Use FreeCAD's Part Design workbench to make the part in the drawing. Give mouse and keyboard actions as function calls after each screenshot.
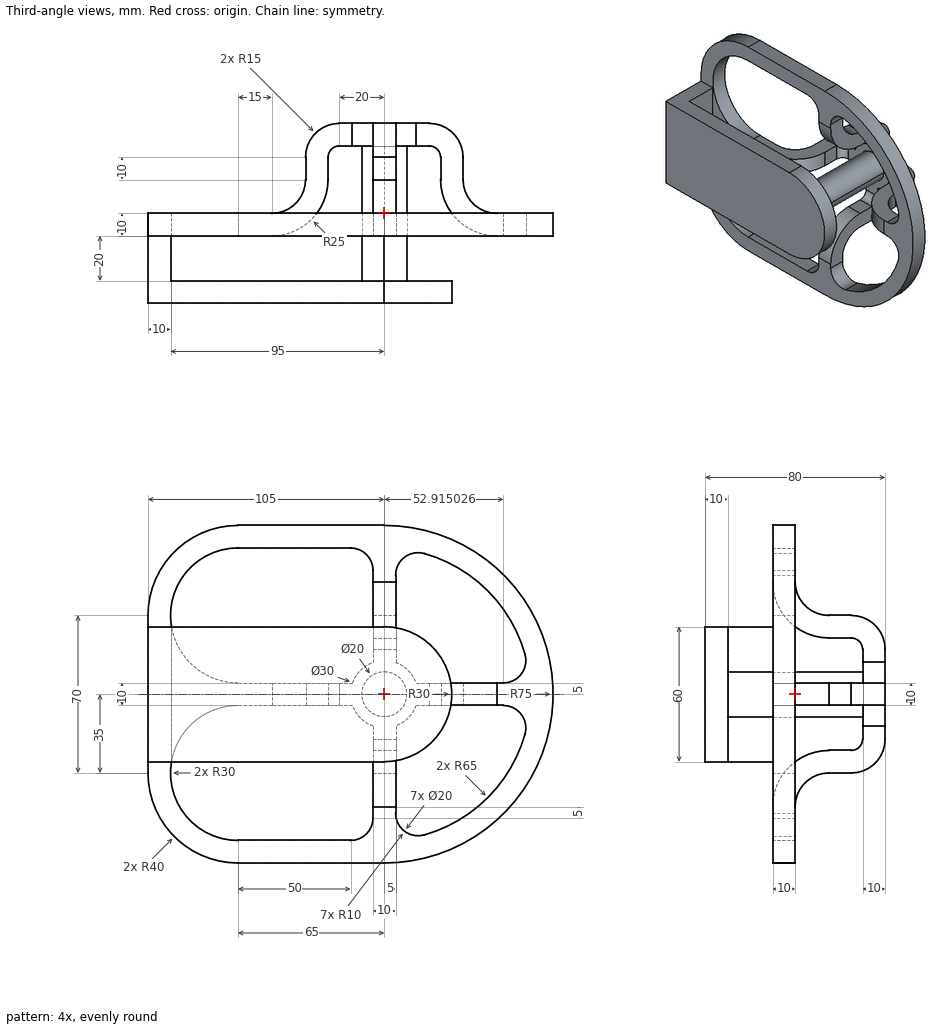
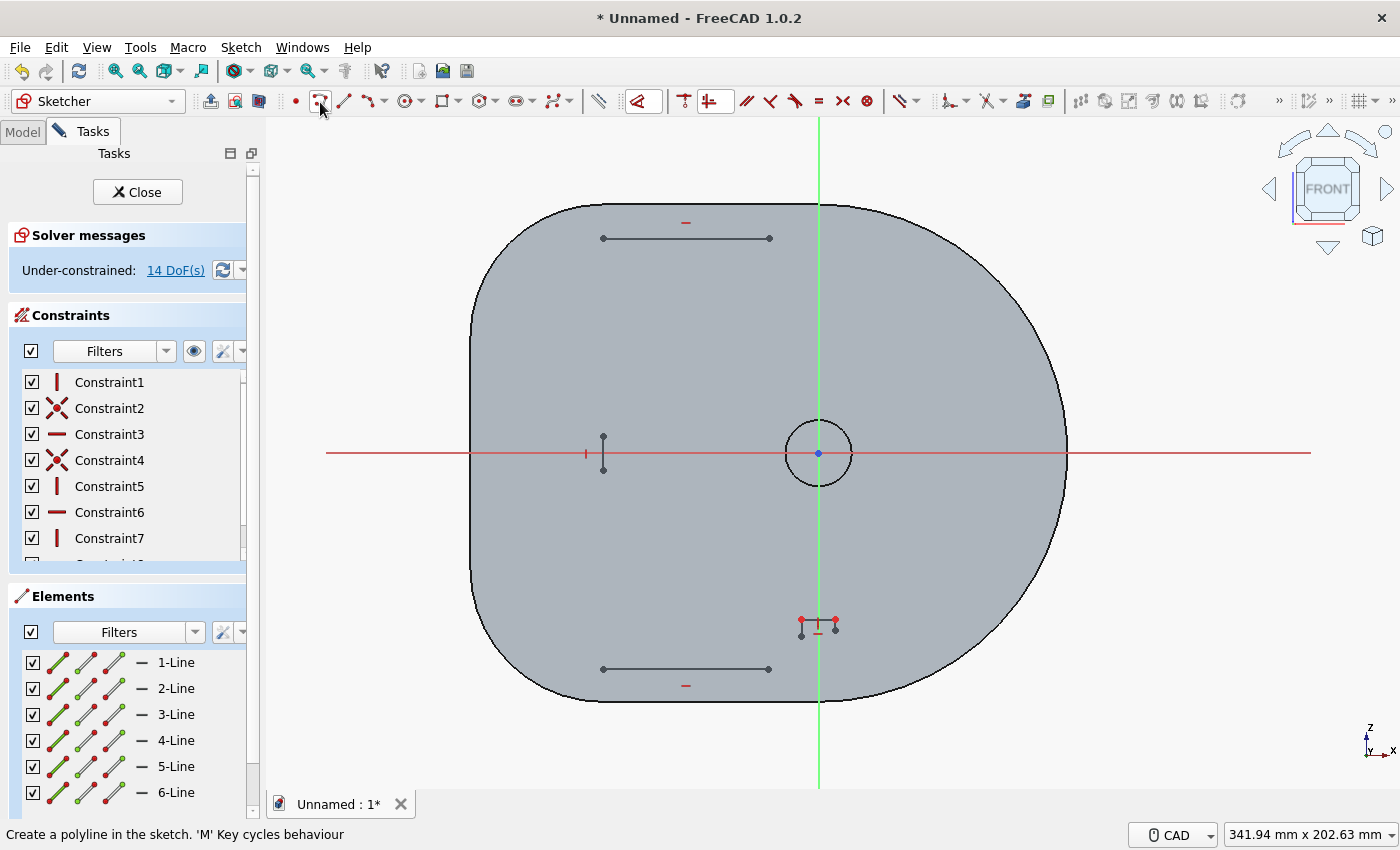
click(802, 271)
click(802, 287)
click(835, 287)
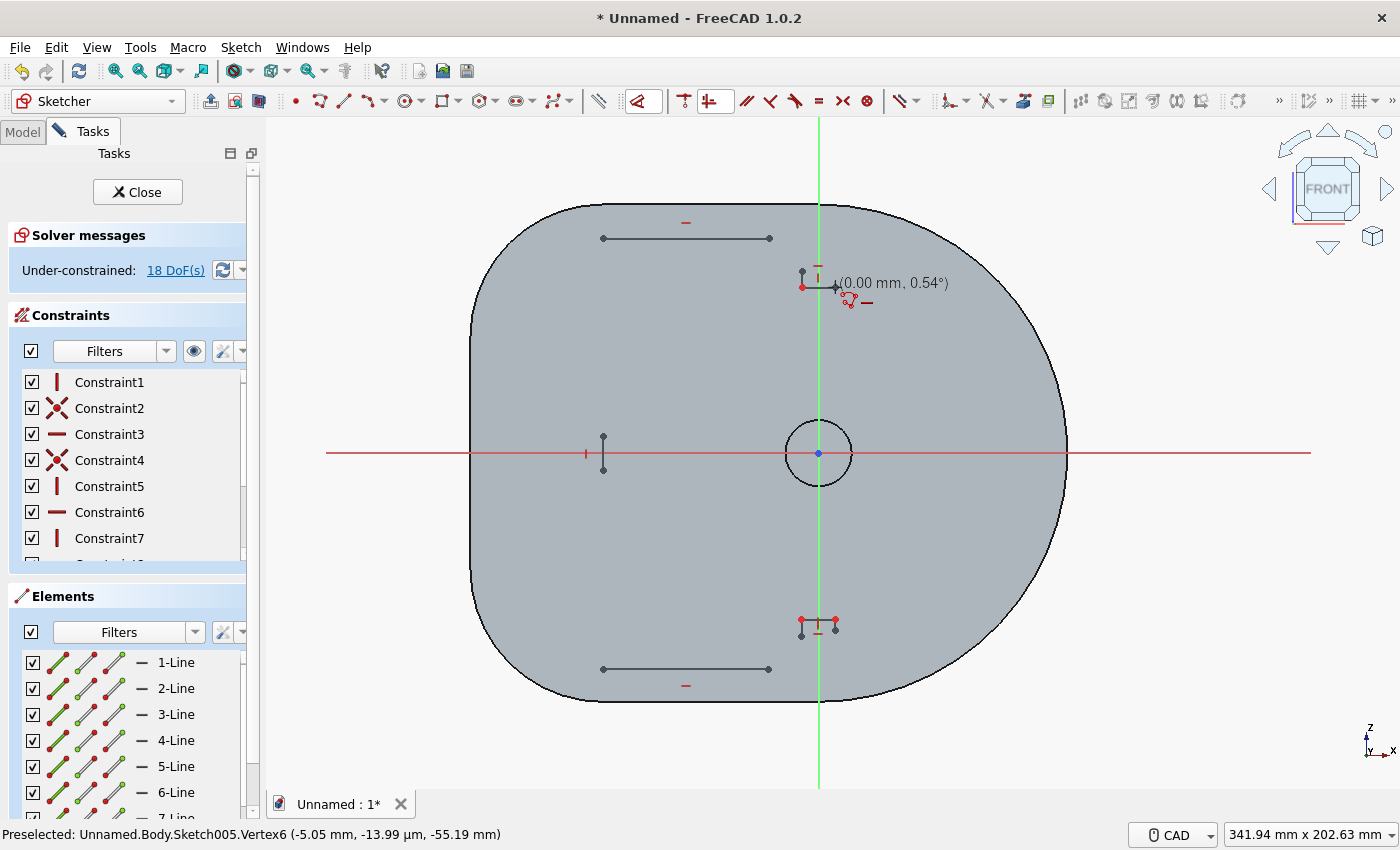
scroll(835, 278, up, 3)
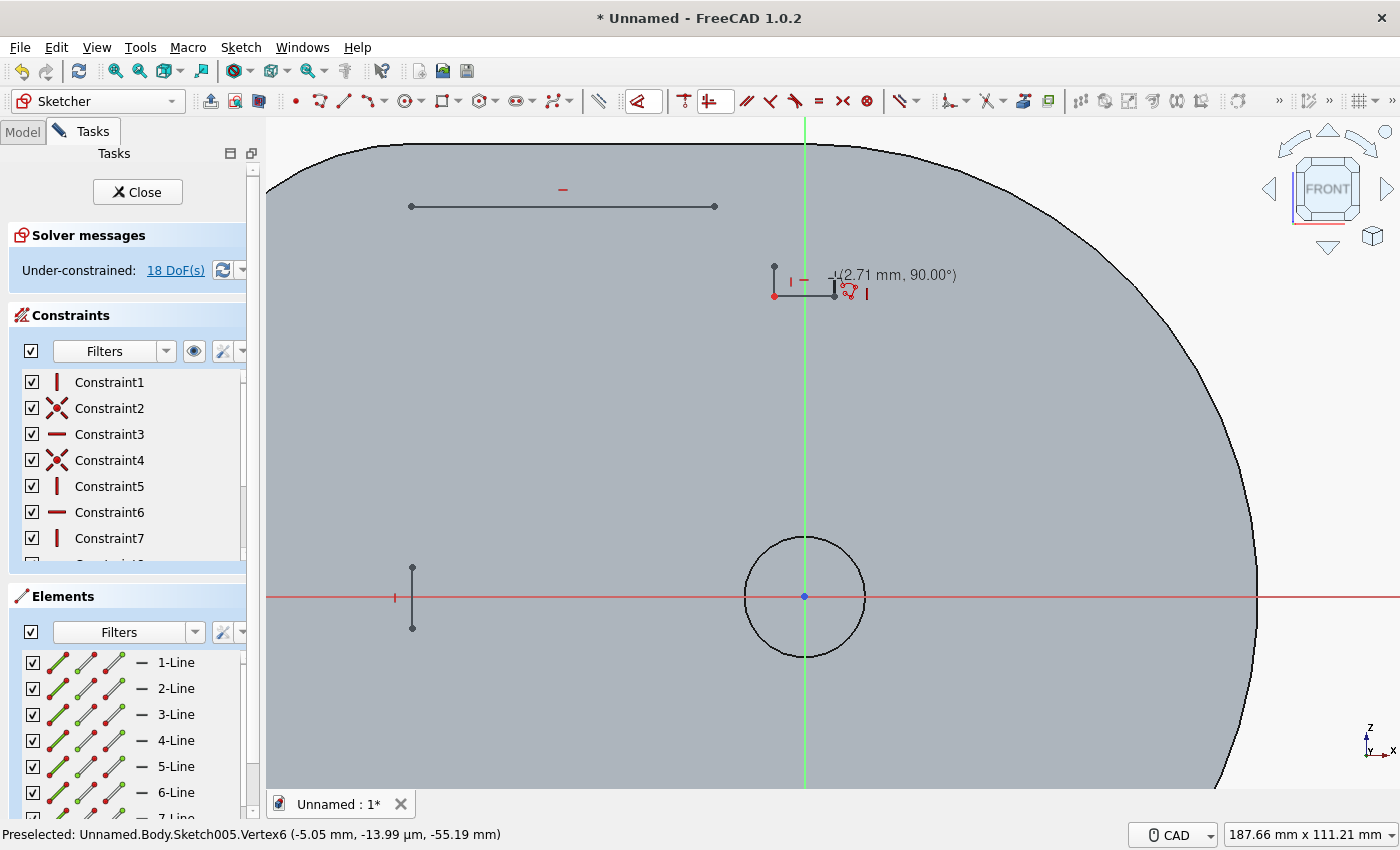
click(835, 277)
right_click(835, 277)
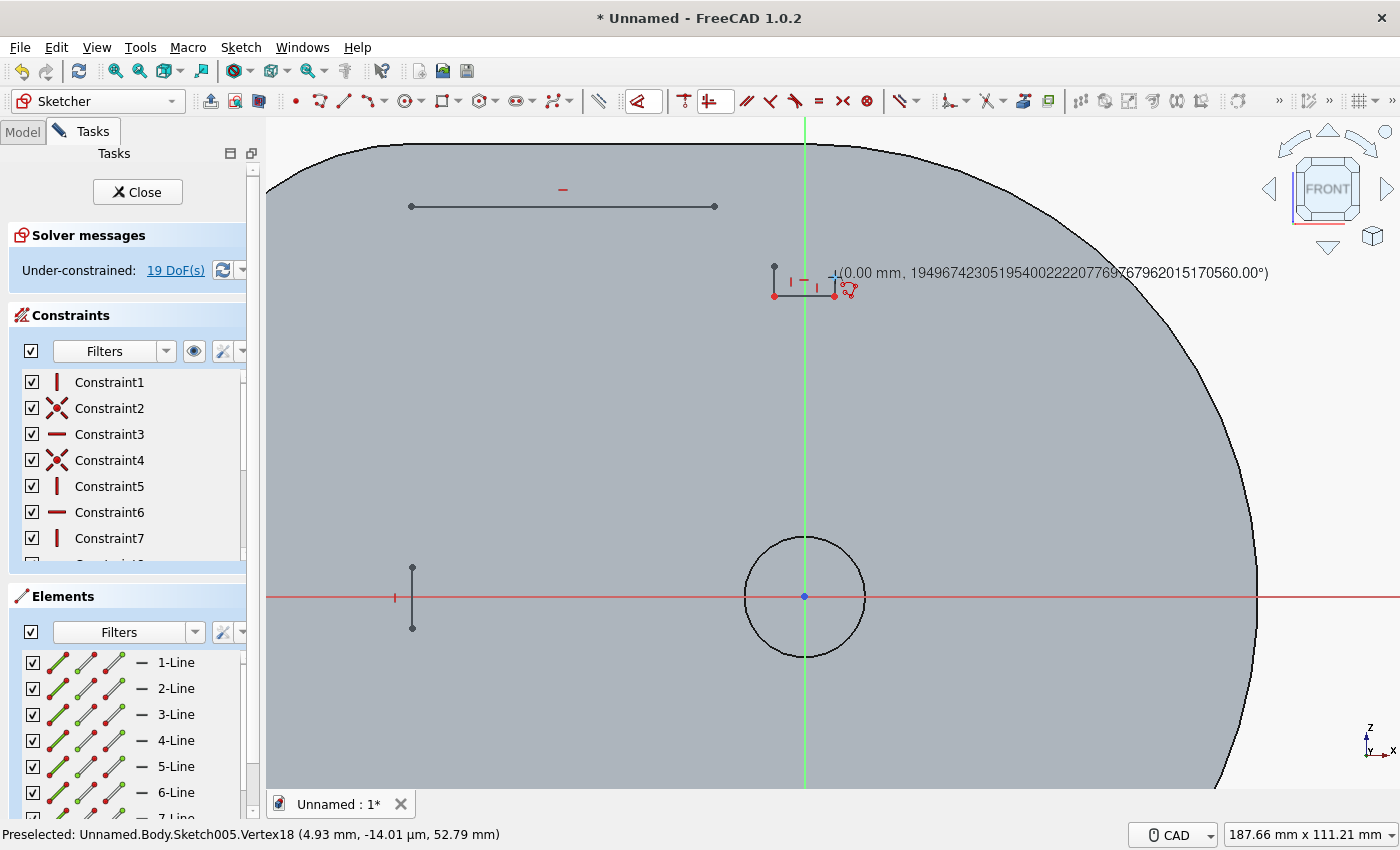
click(344, 102)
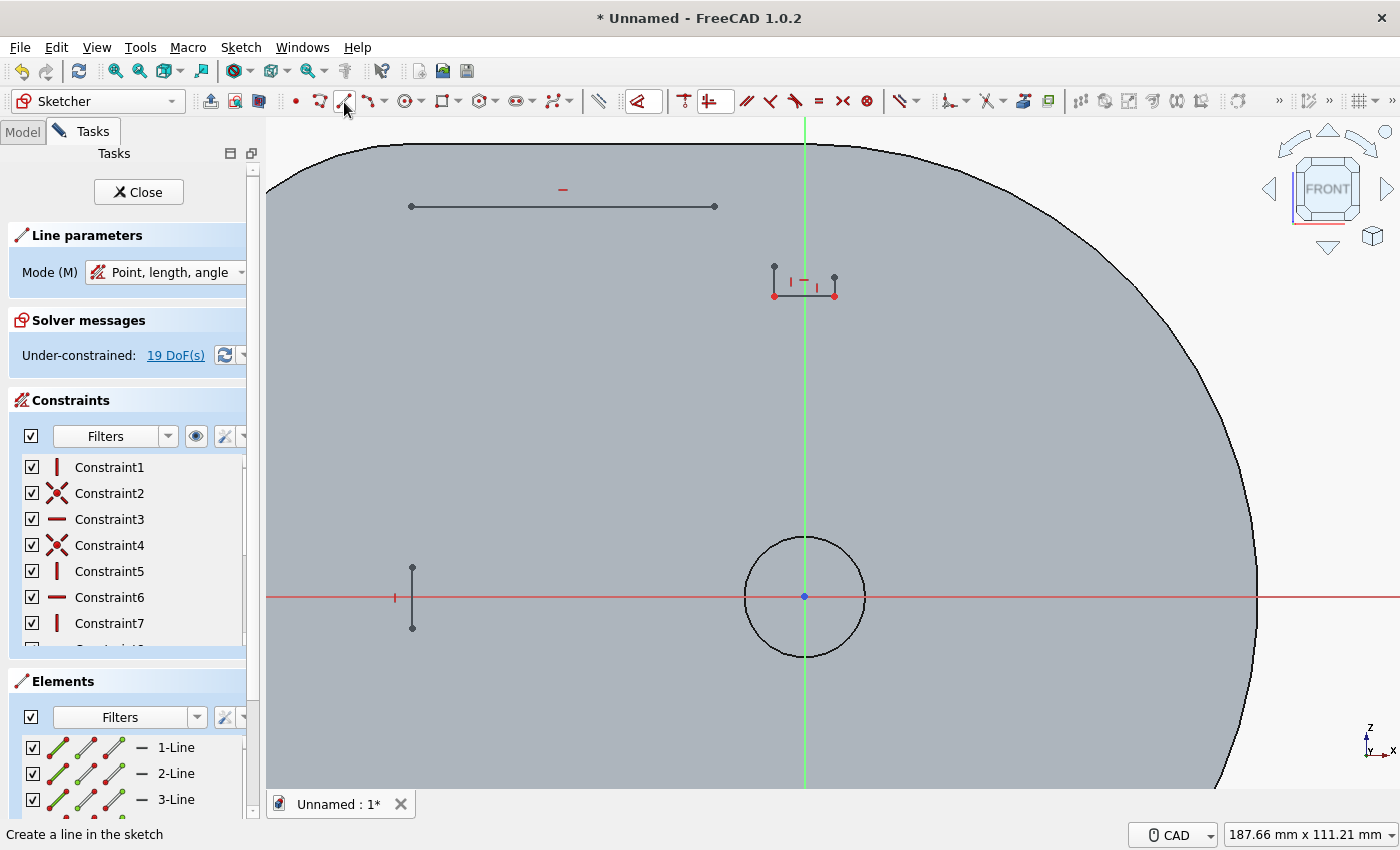
click(1125, 567)
click(1125, 627)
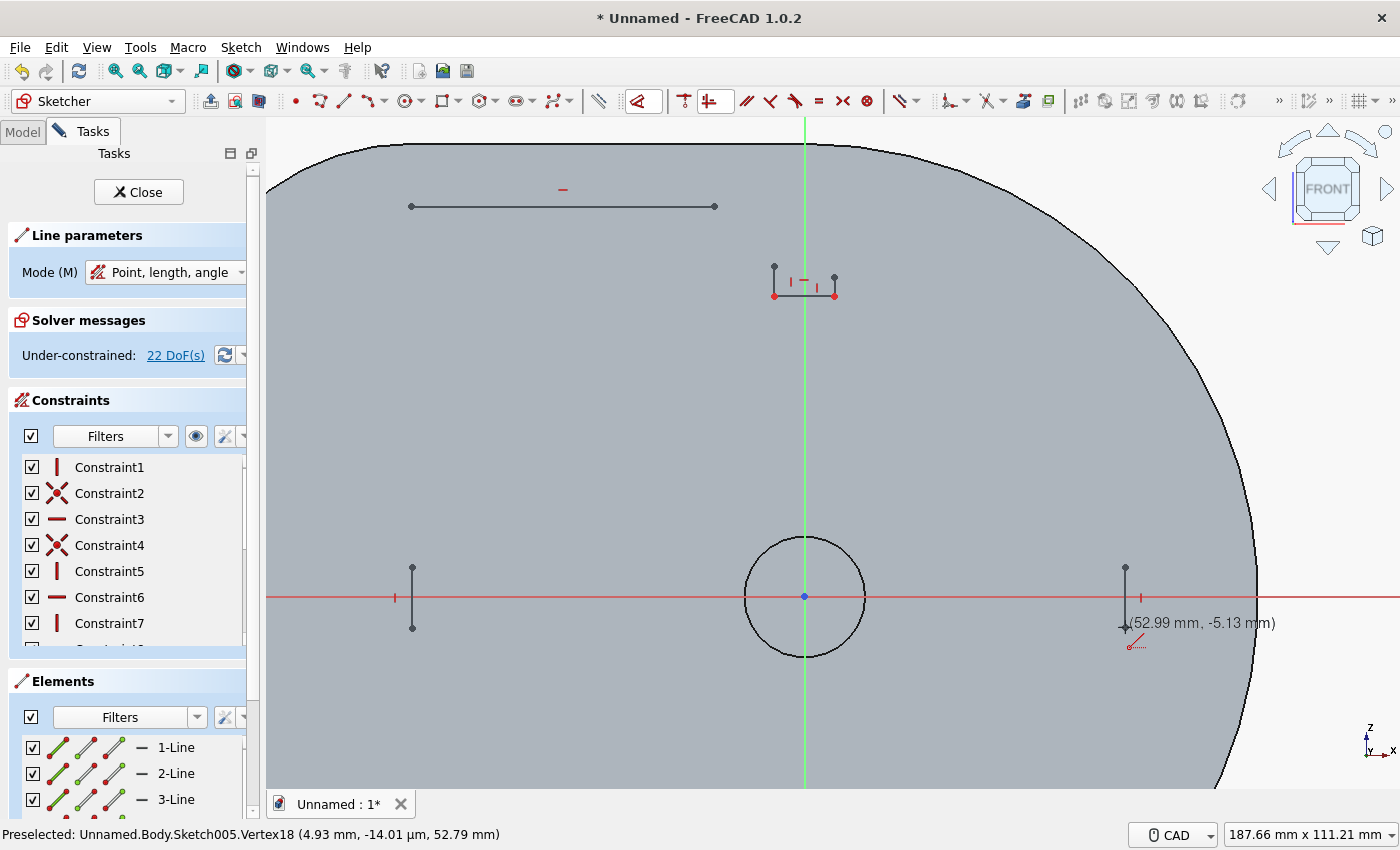
click(368, 102)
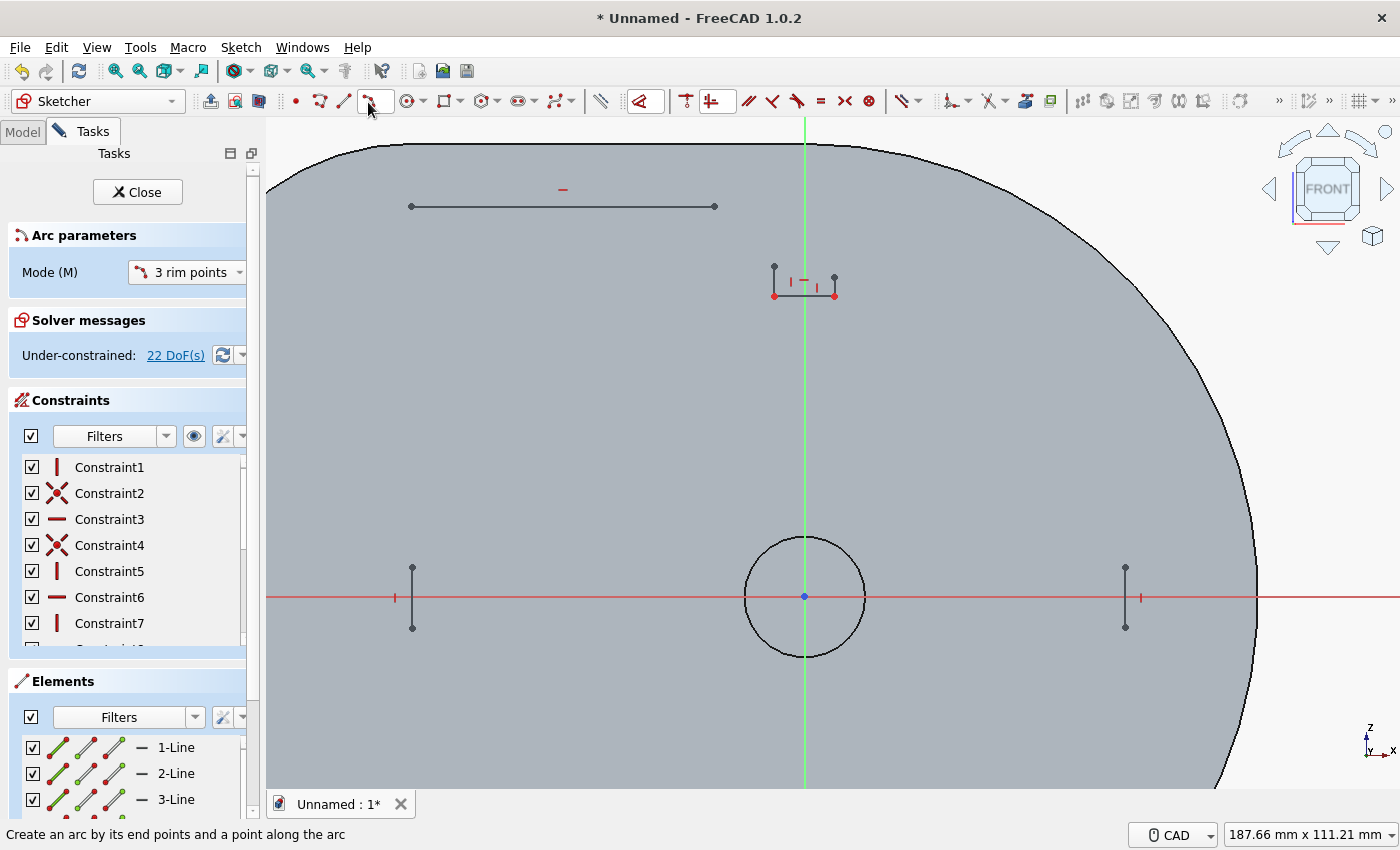
scroll(835, 278, down, 3)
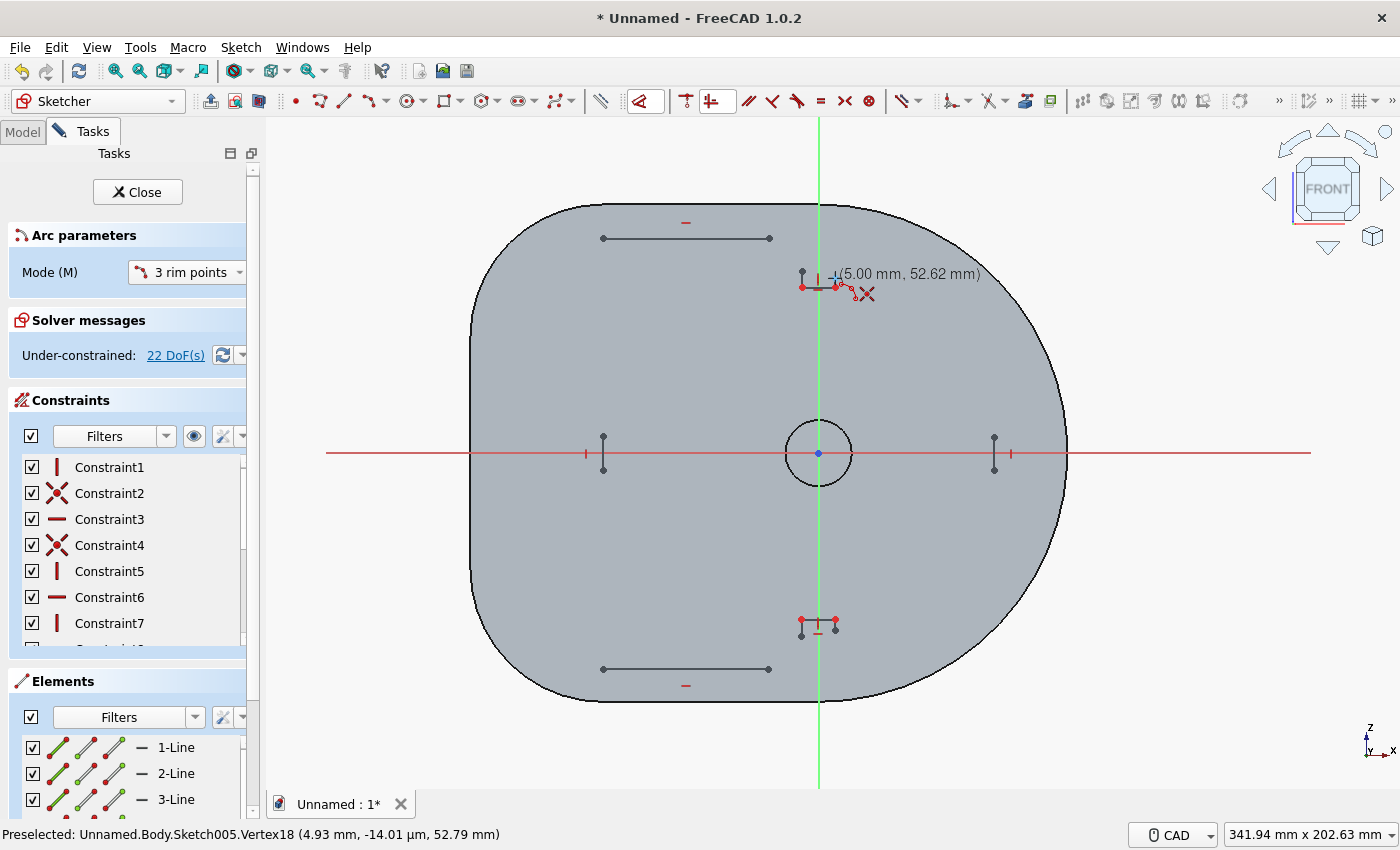
scroll(802, 636, up, 4)